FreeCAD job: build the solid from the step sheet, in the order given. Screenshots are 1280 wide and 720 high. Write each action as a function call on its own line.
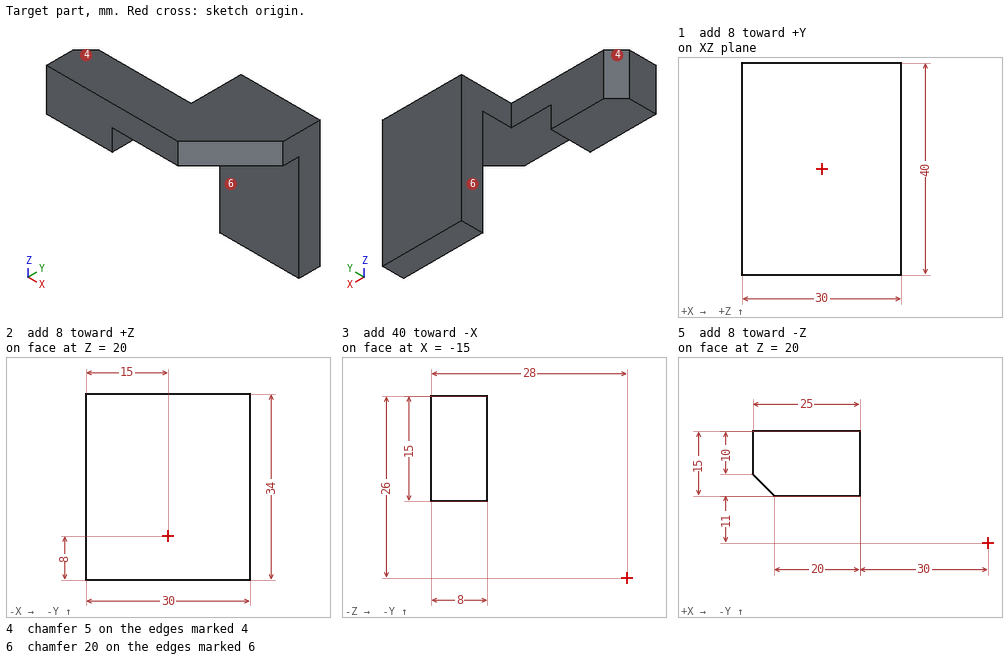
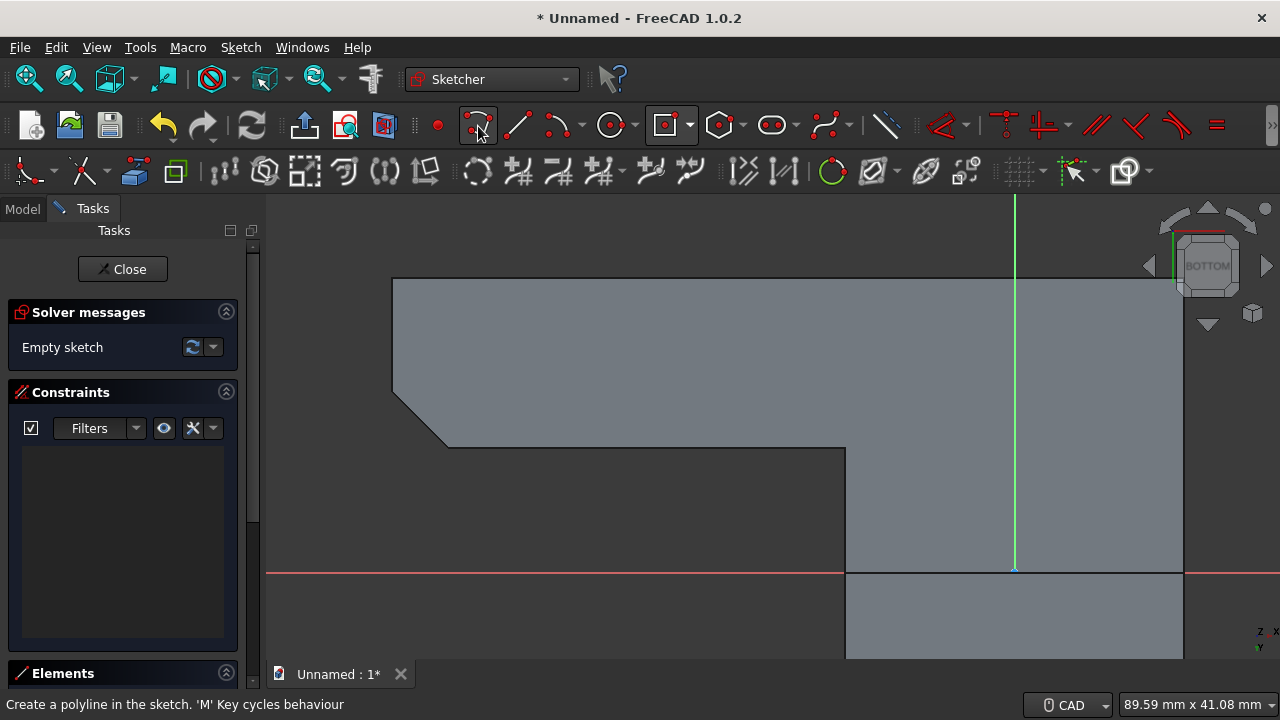
click(675, 448)
click(675, 278)
click(392, 278)
click(392, 391)
click(449, 448)
click(675, 449)
key(Escape)
key(Escape)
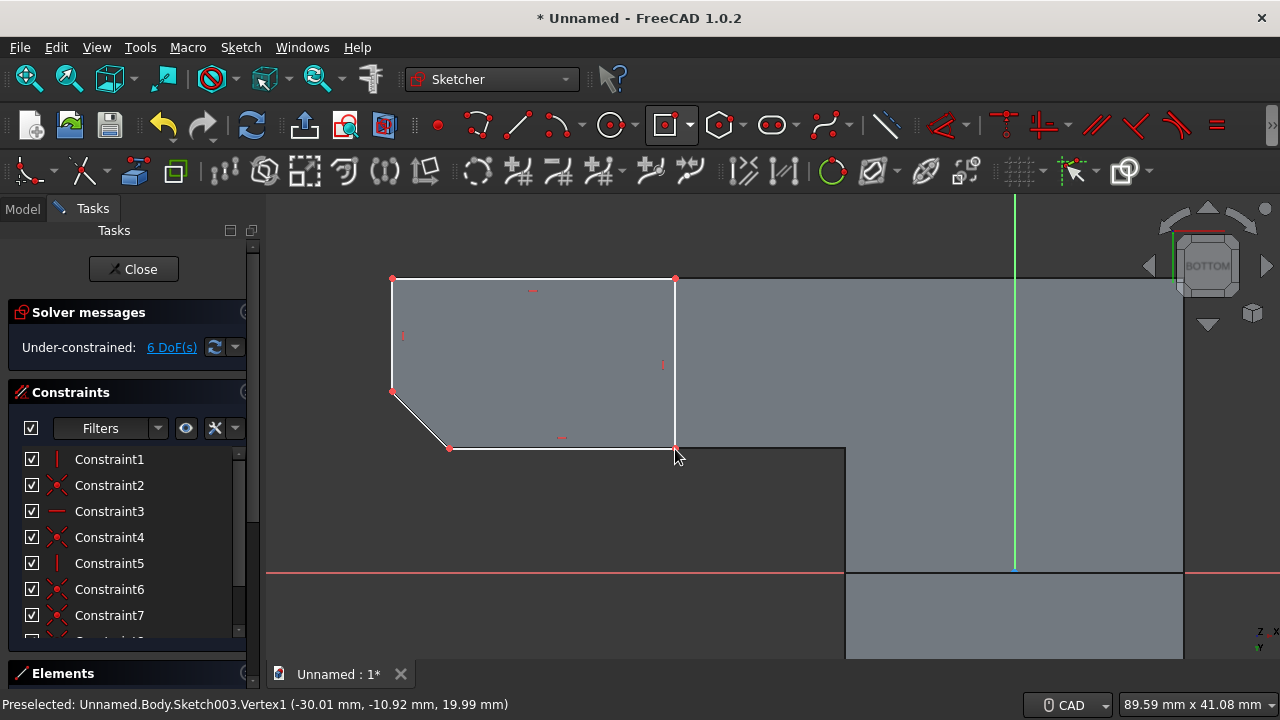
click(942, 126)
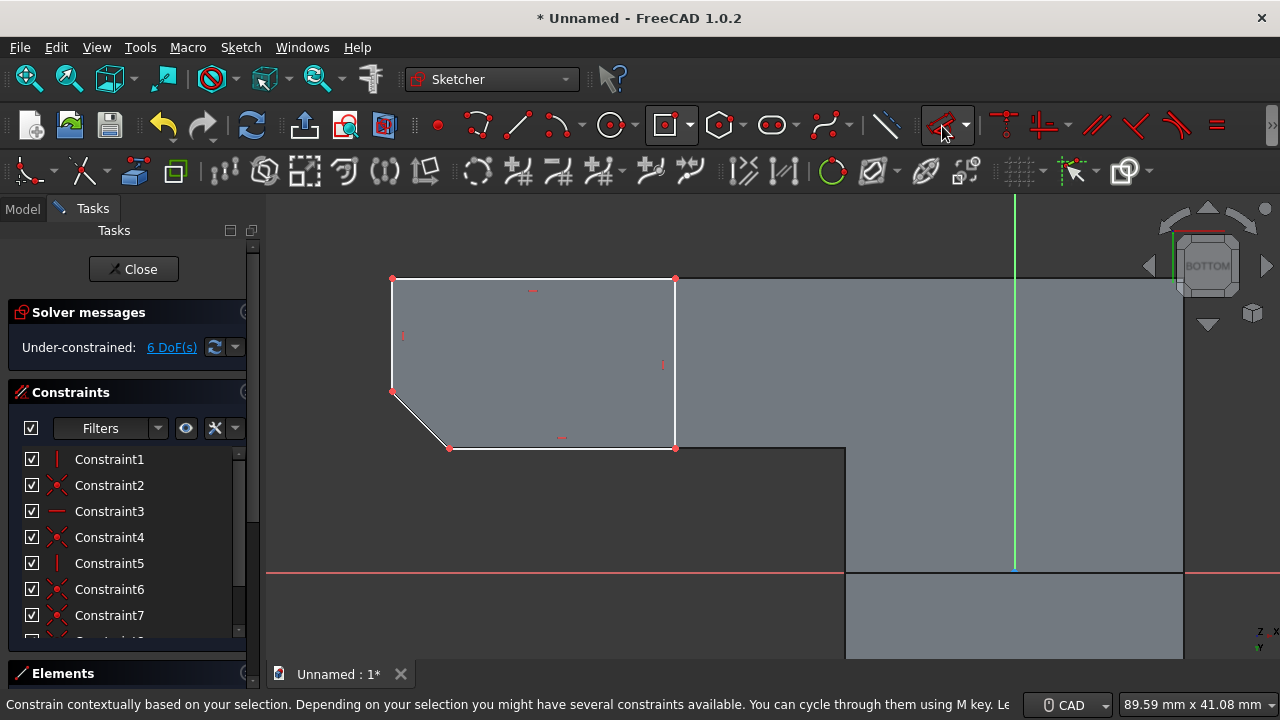
click(675, 398)
click(641, 364)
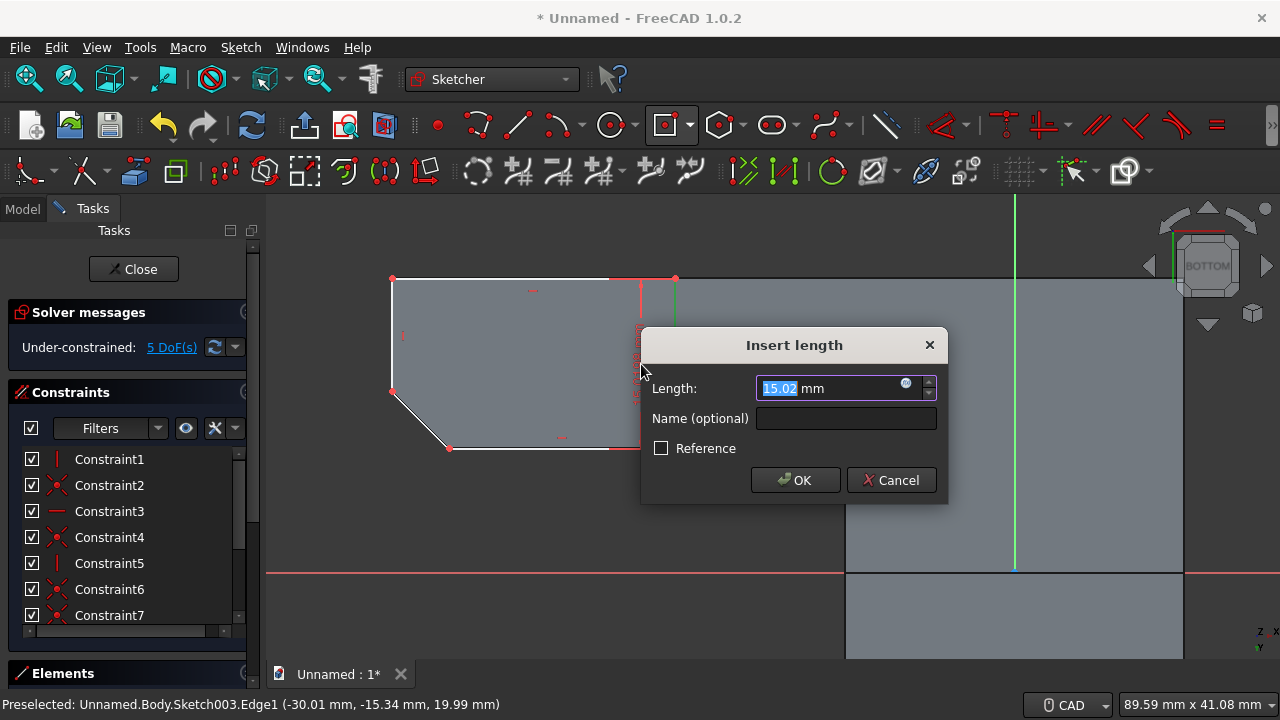
text(15)
key(Return)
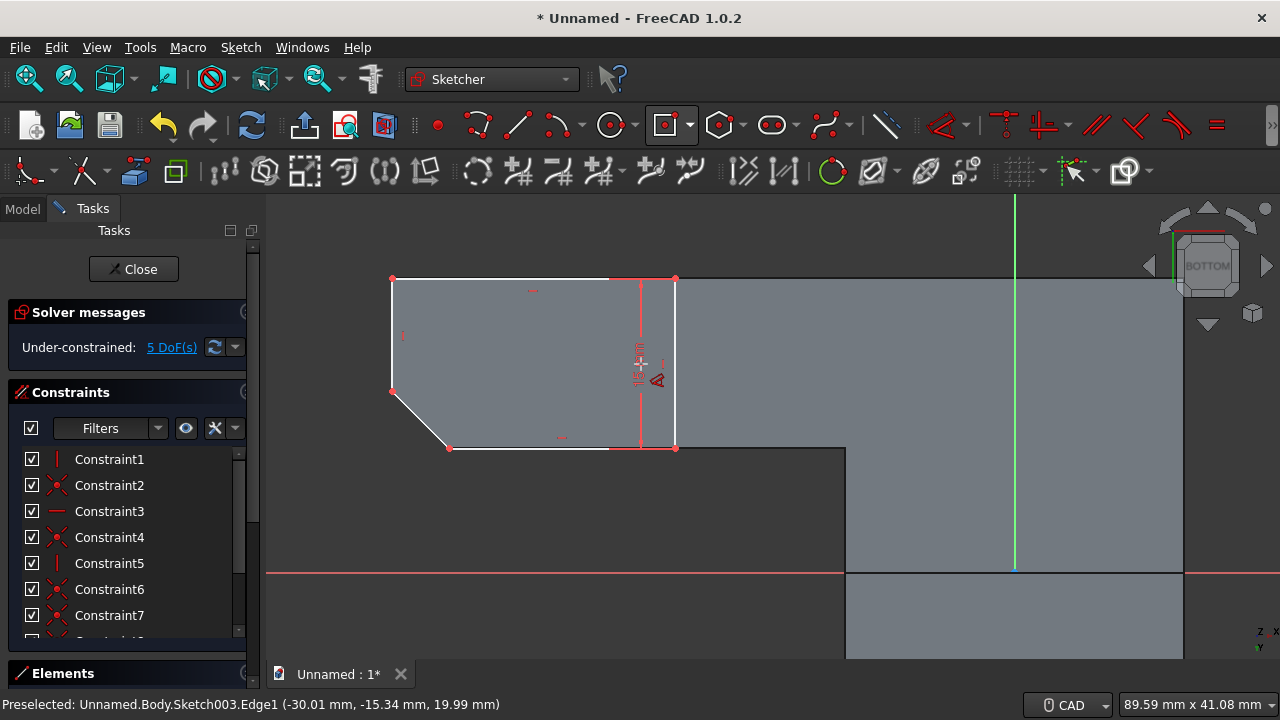
click(590, 279)
click(533, 245)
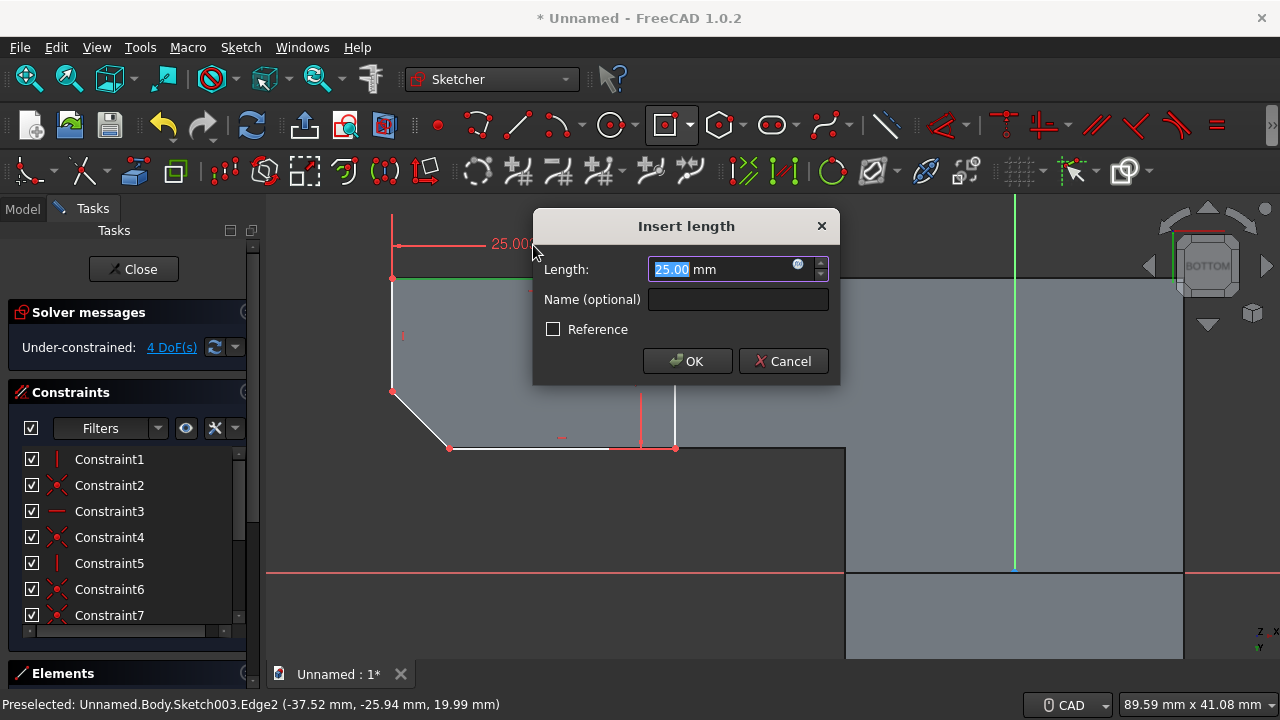
text(25)
key(Return)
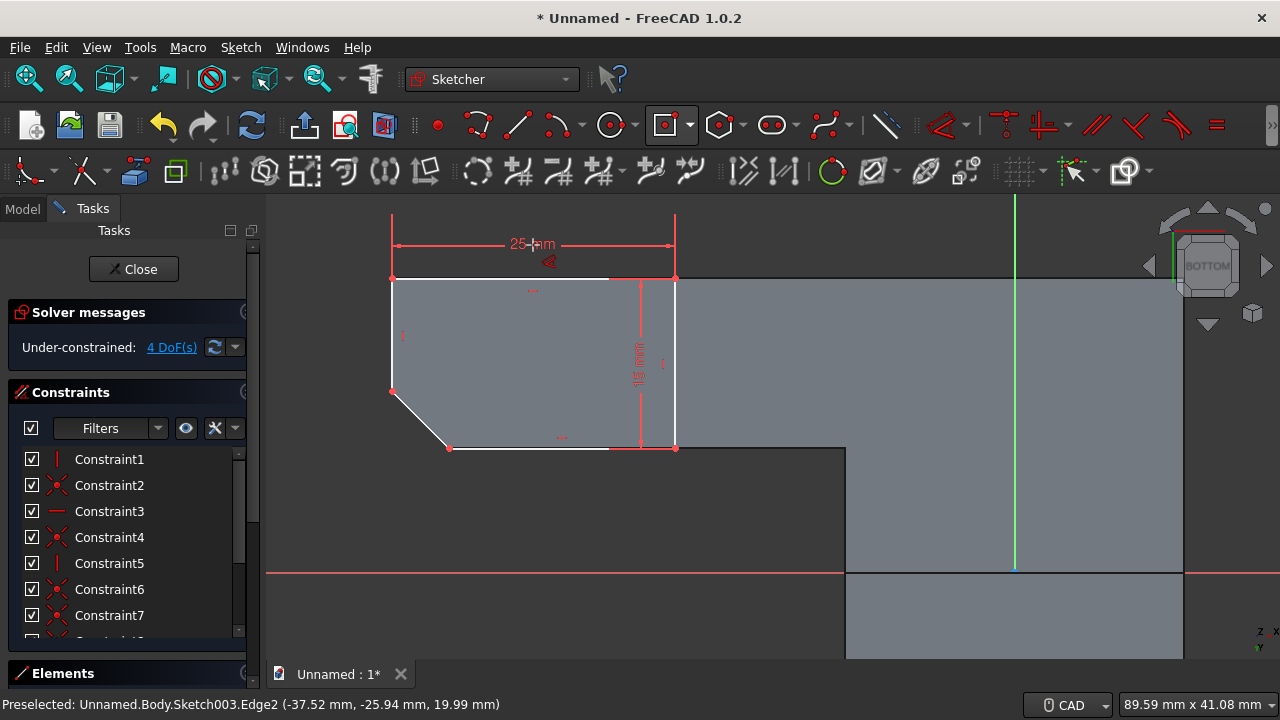
click(392, 313)
click(358, 336)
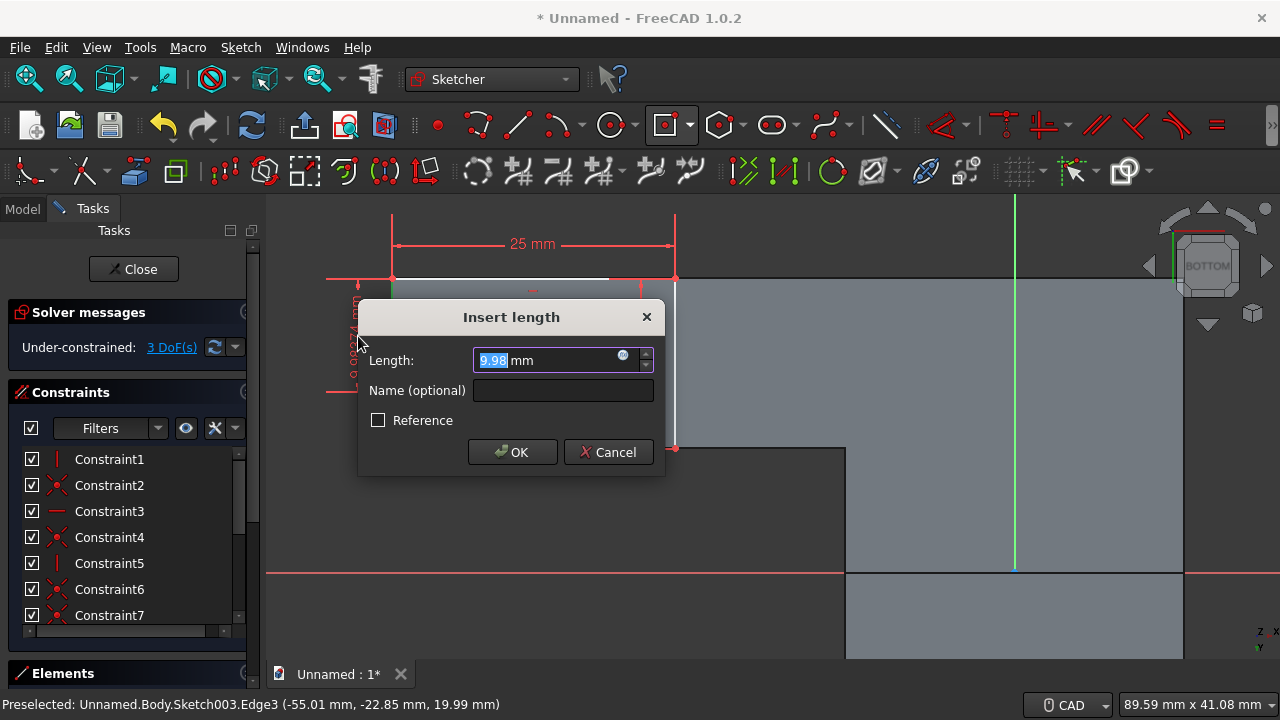
text(10)
key(Return)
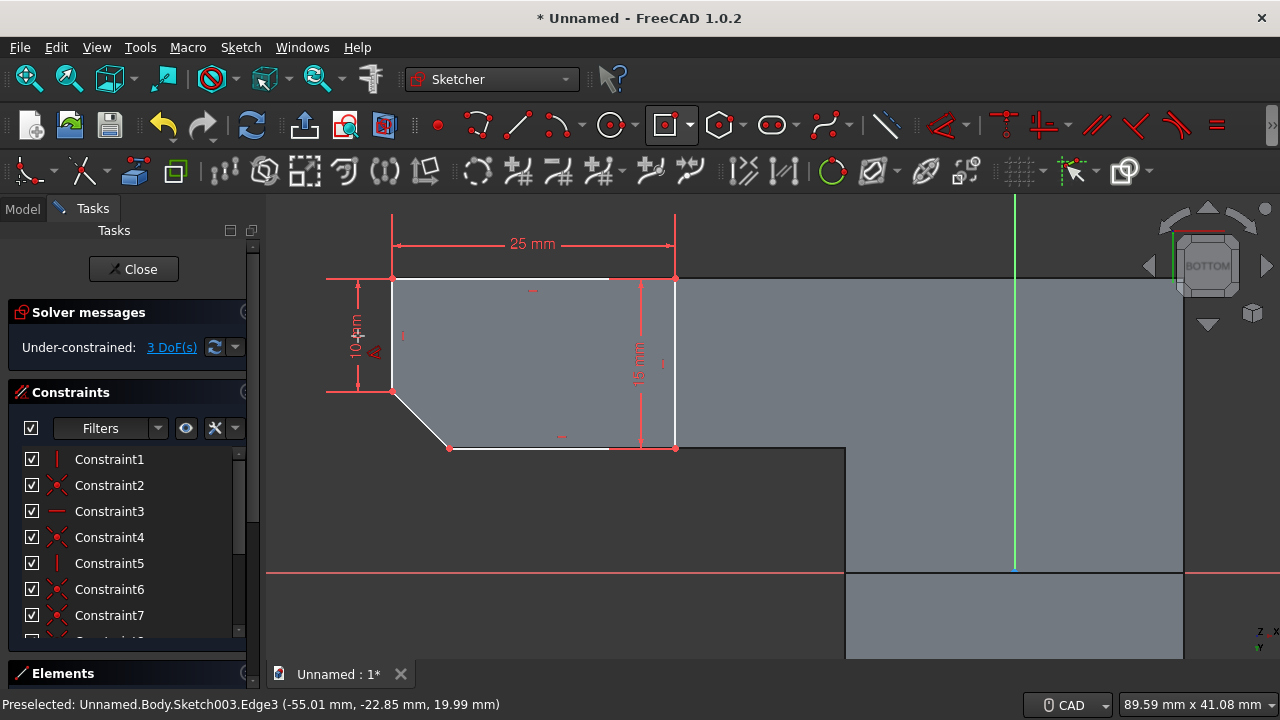
click(517, 449)
click(562, 483)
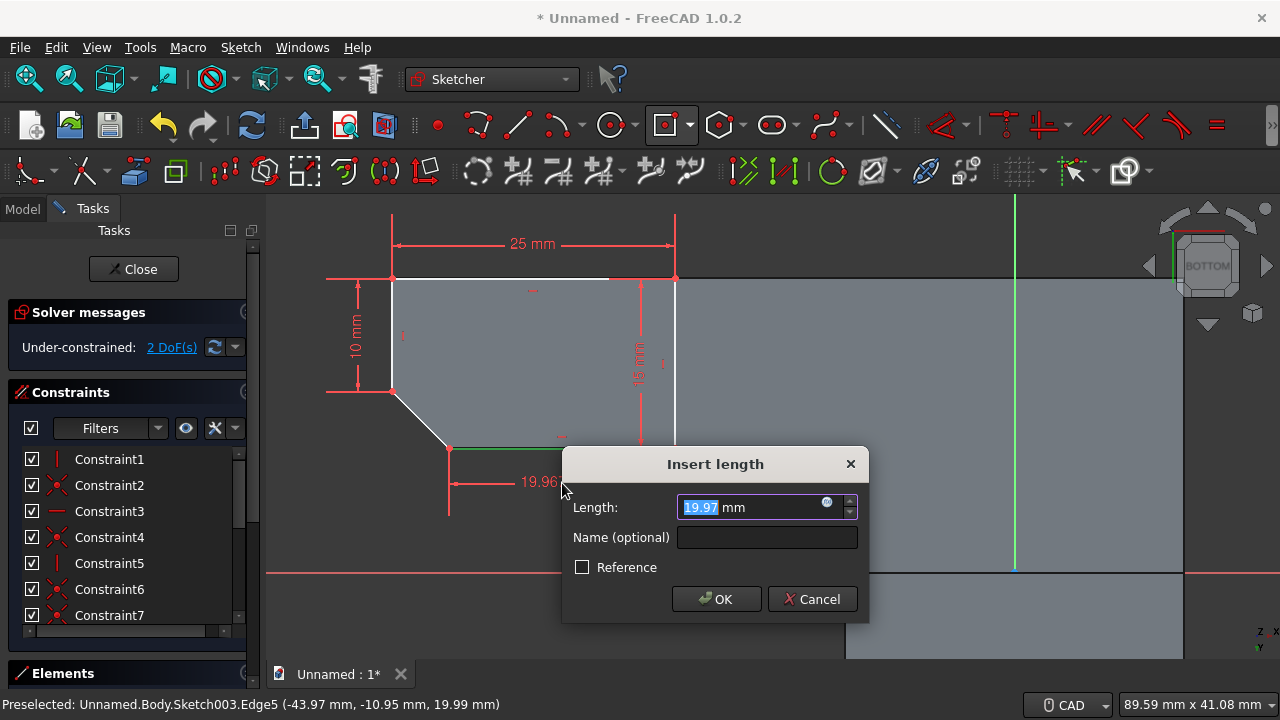
text(20)
key(Return)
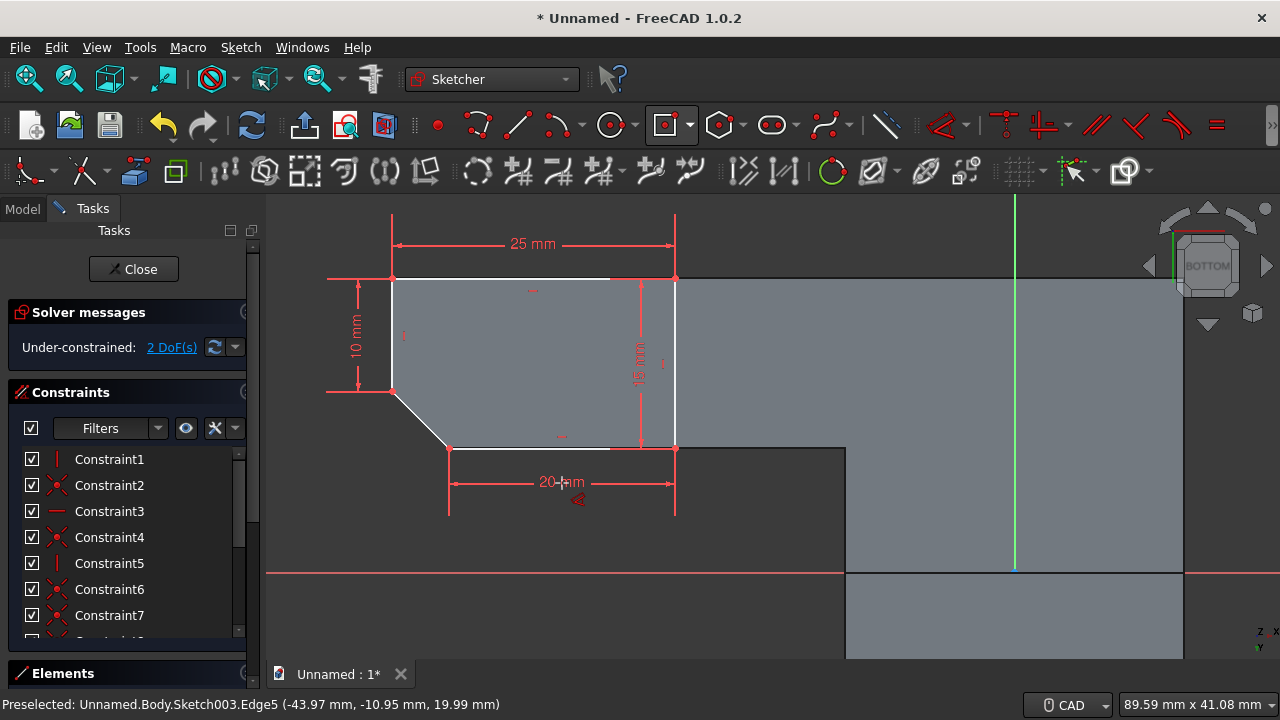
click(675, 449)
click(845, 607)